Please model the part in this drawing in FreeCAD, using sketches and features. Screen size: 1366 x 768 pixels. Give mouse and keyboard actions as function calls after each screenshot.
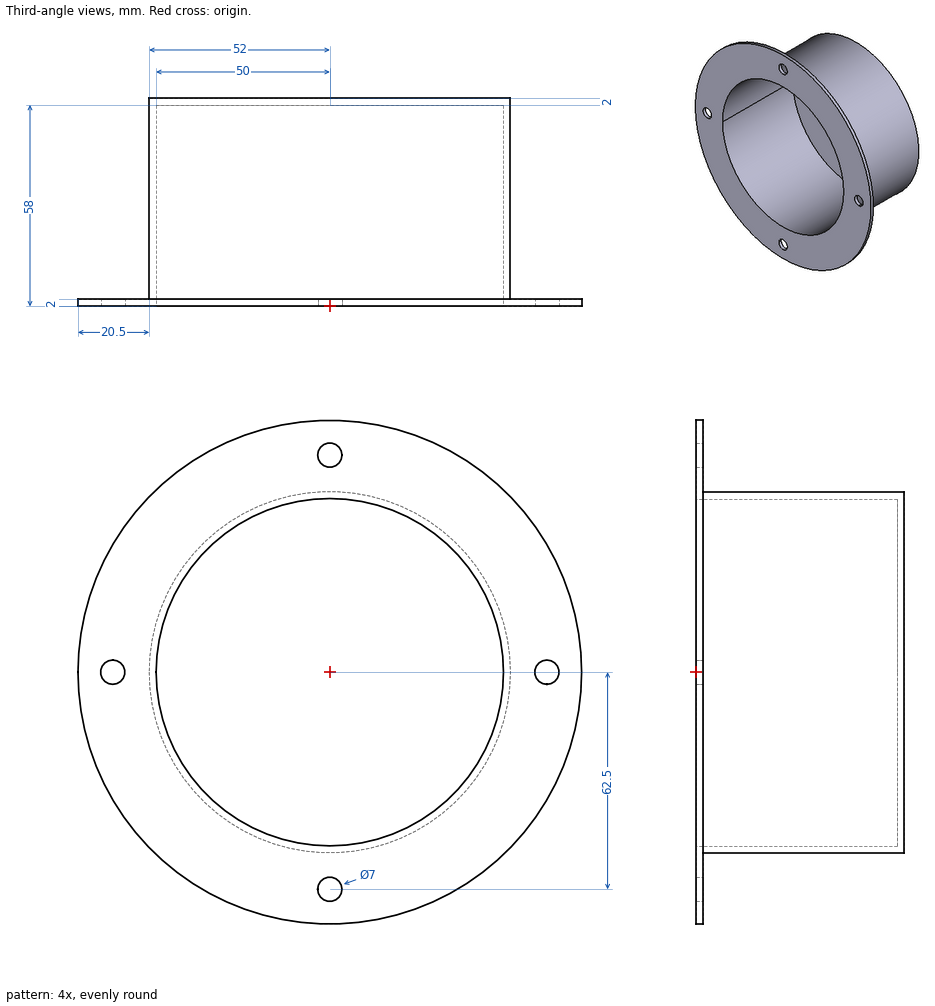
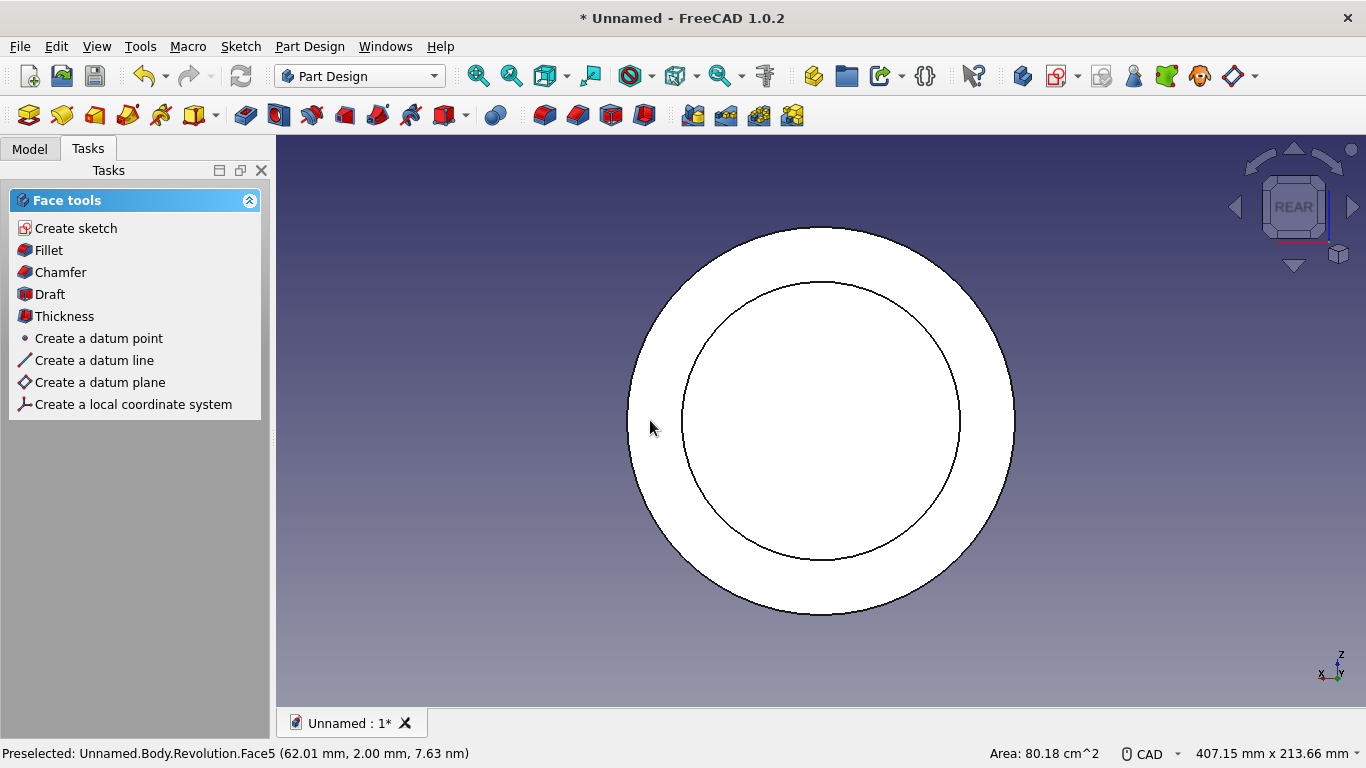
click(1056, 76)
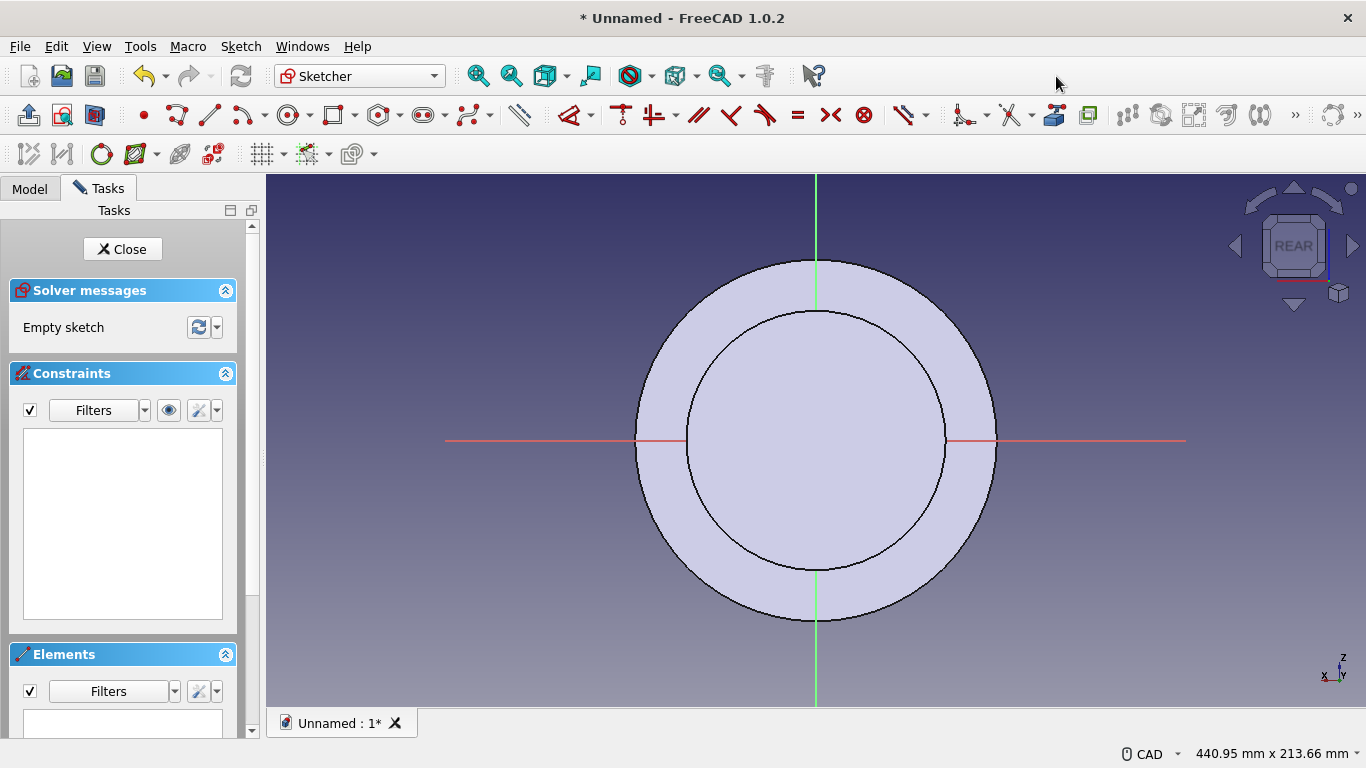
key(q)
key(s)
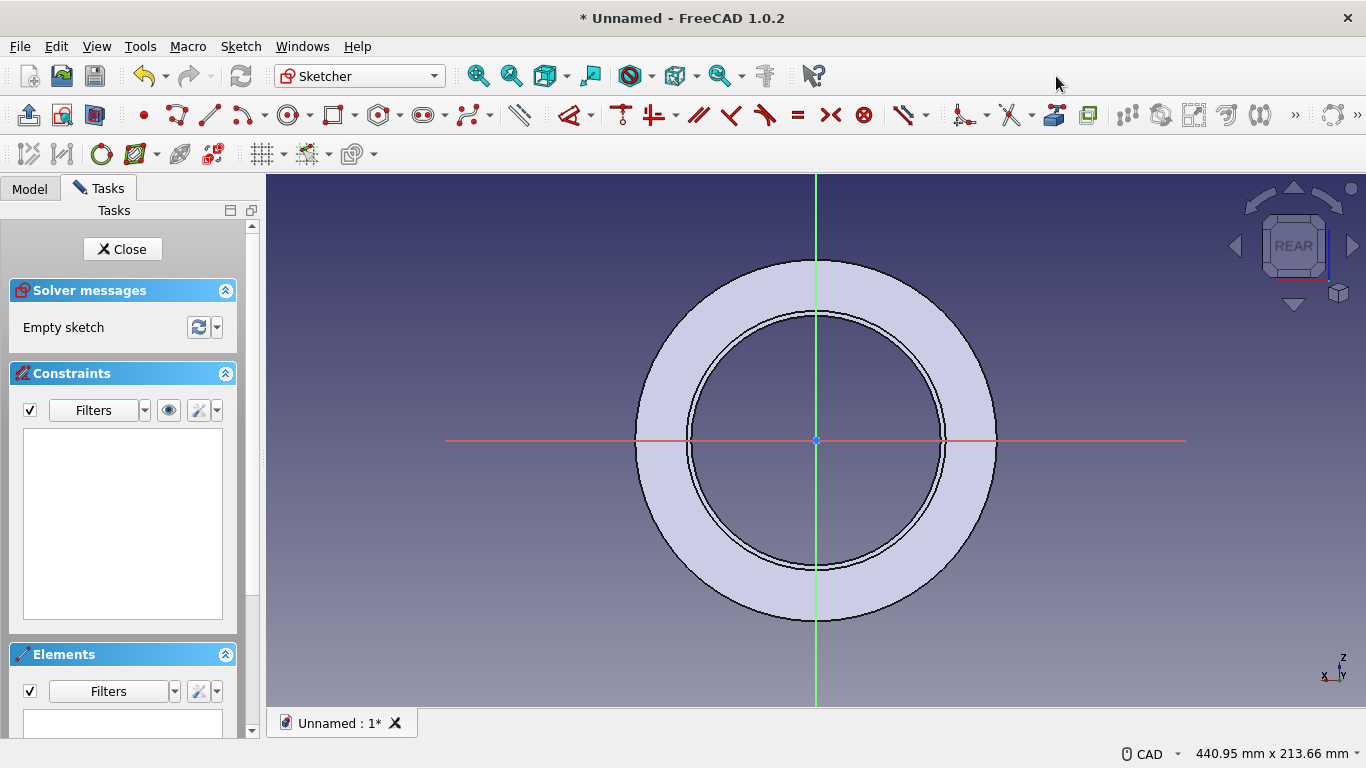
scroll(820, 605, up, 15)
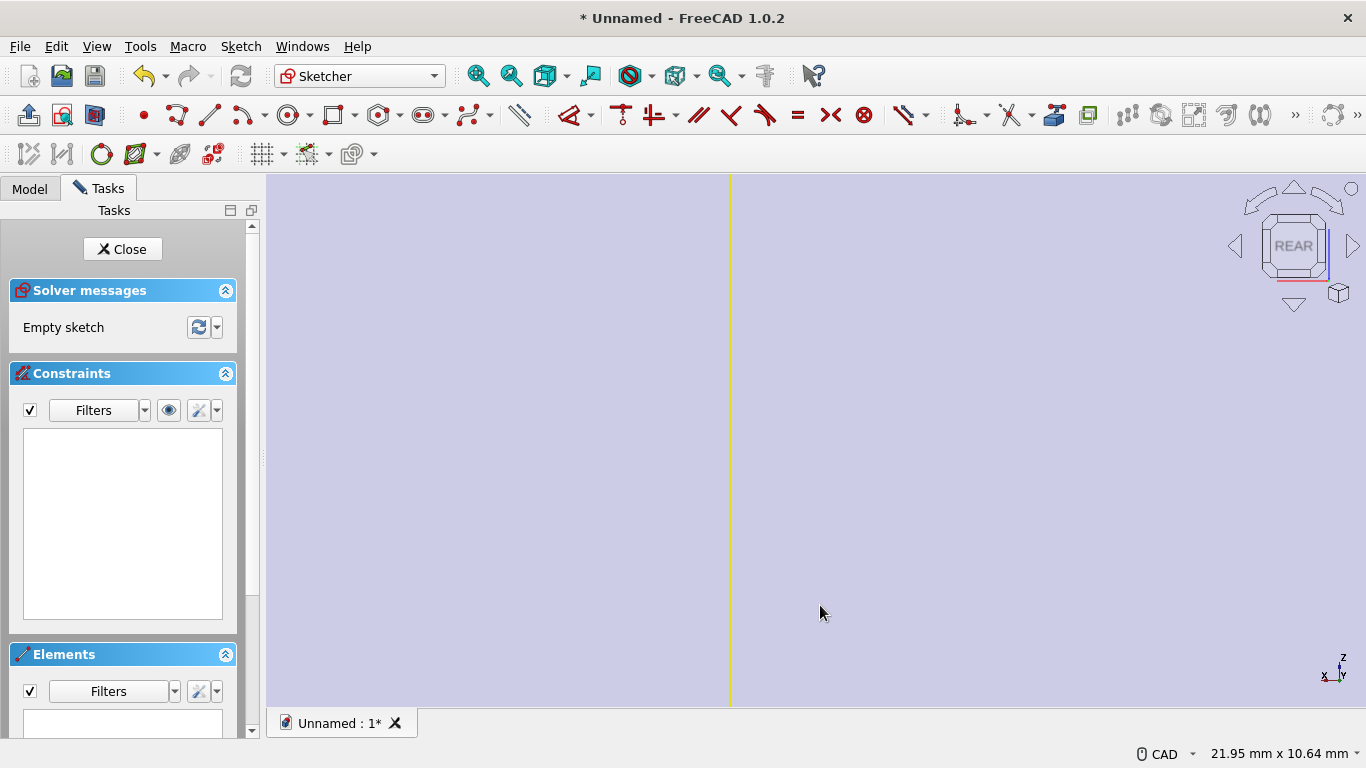
key(g)
key(c)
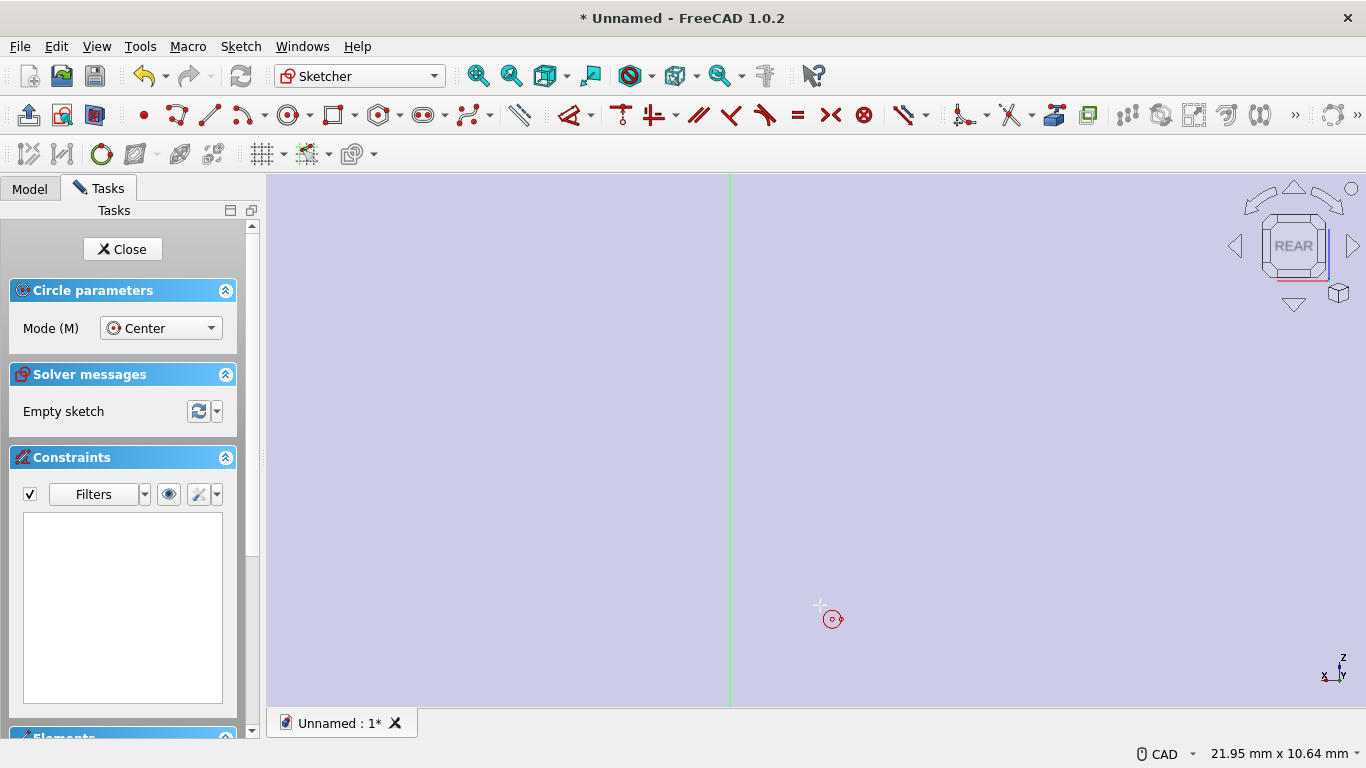
click(730, 417)
move(854, 293)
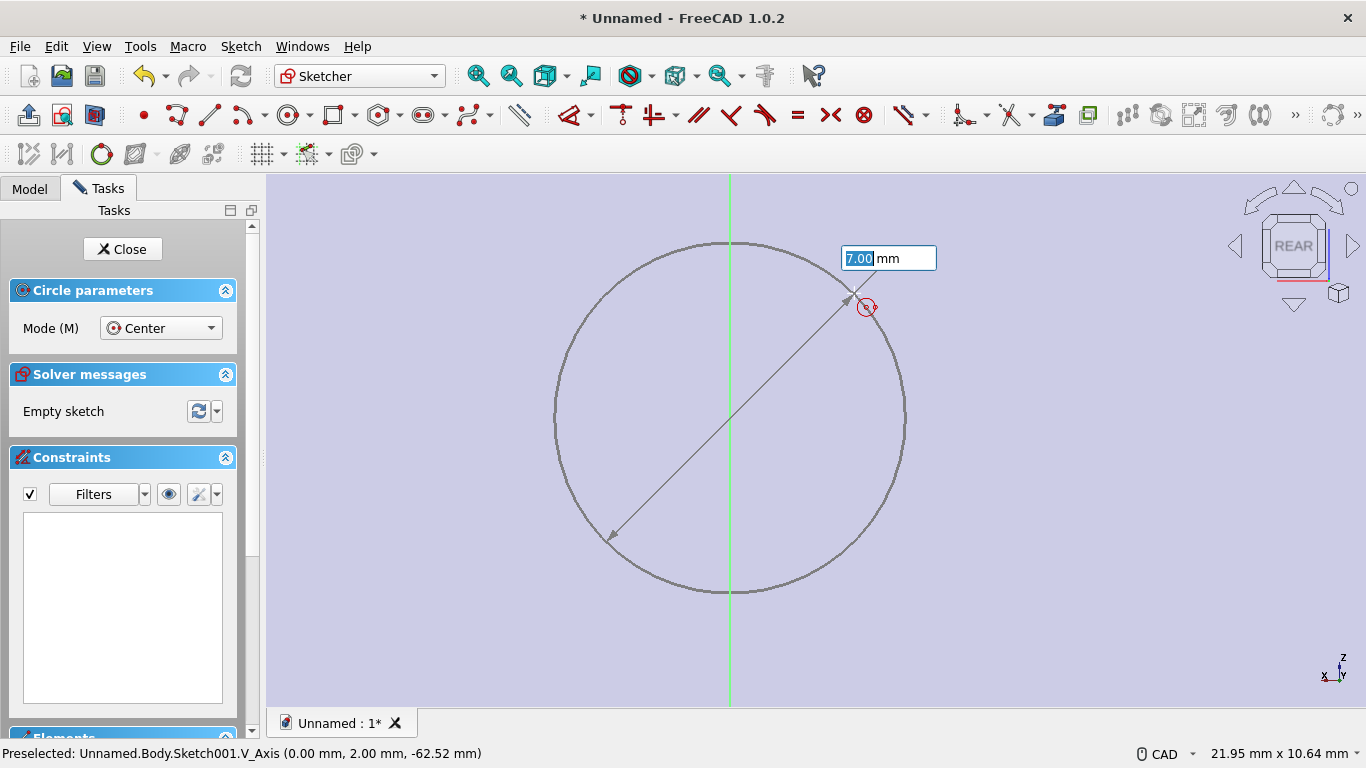
text(7)
key(Return)
key(Escape)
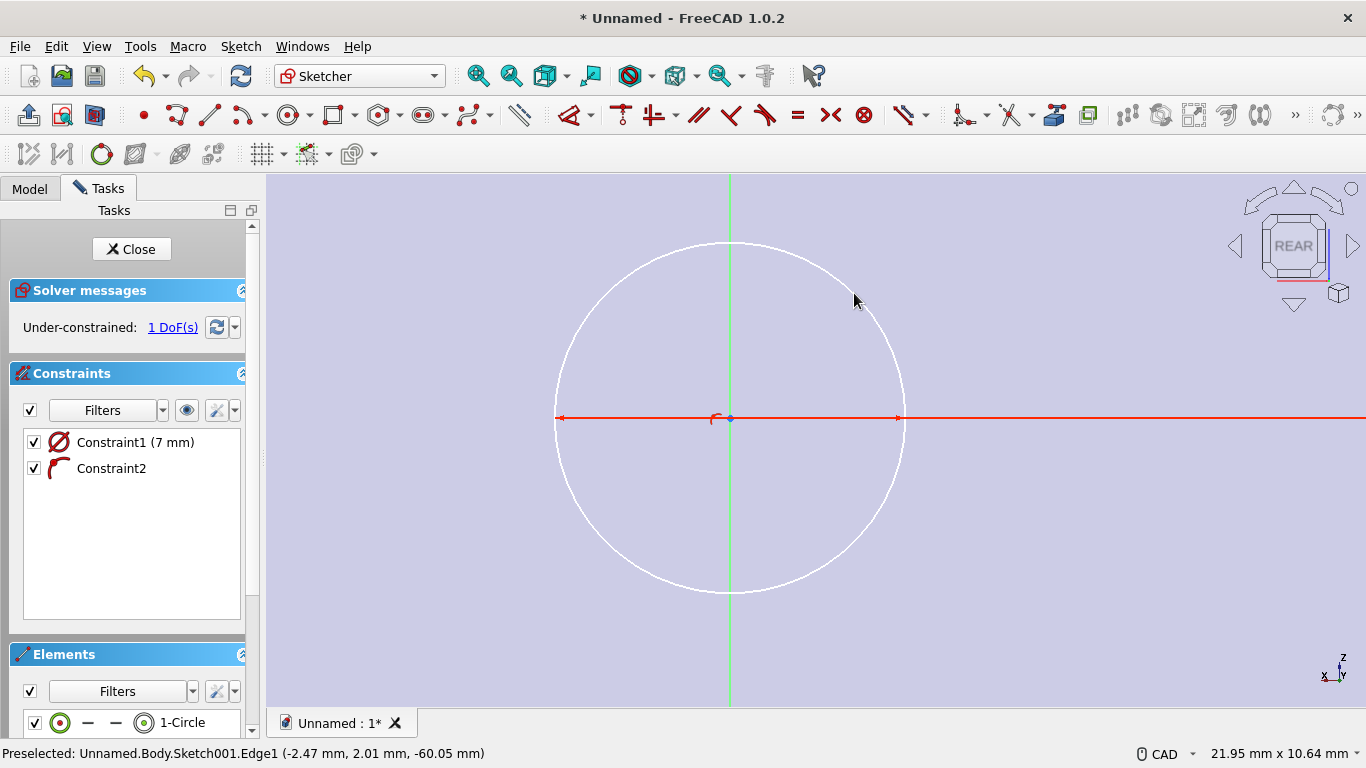
key(d)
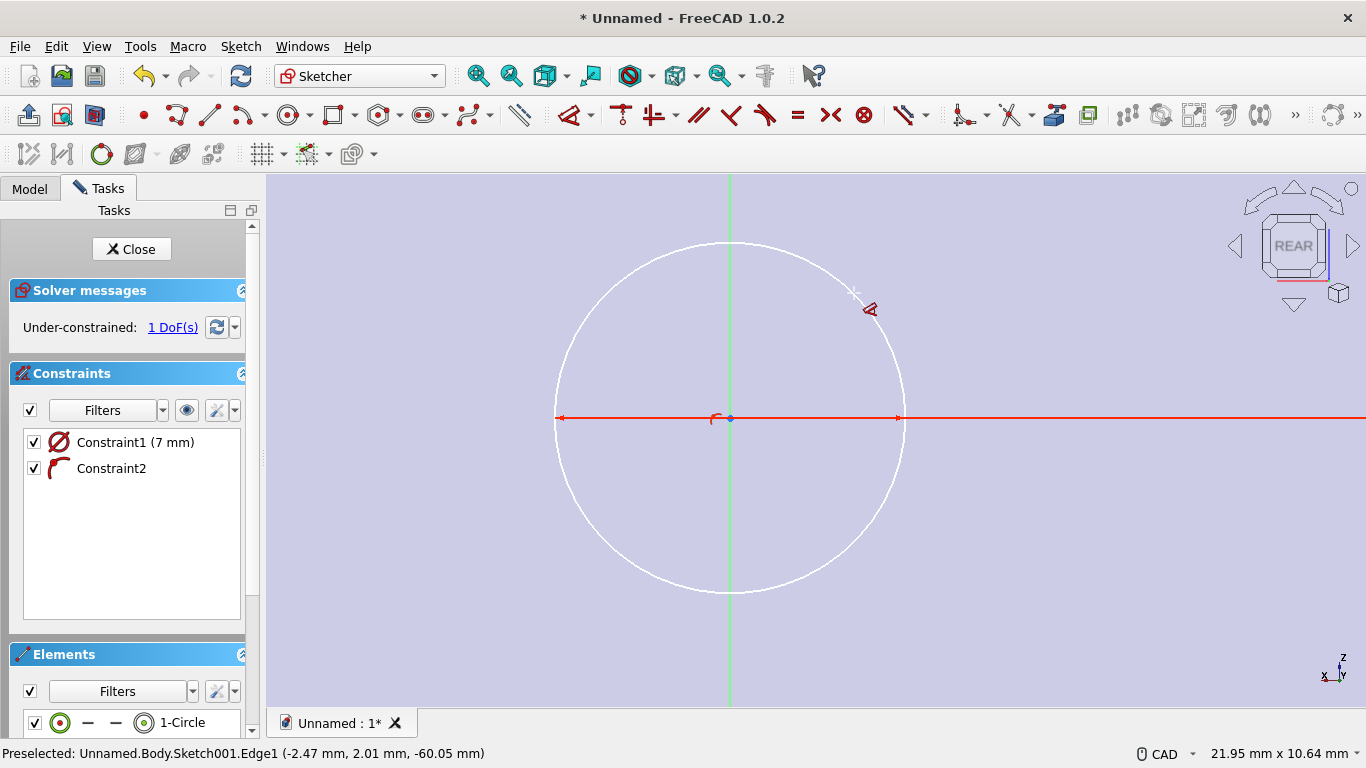
click(730, 418)
click(764, 310)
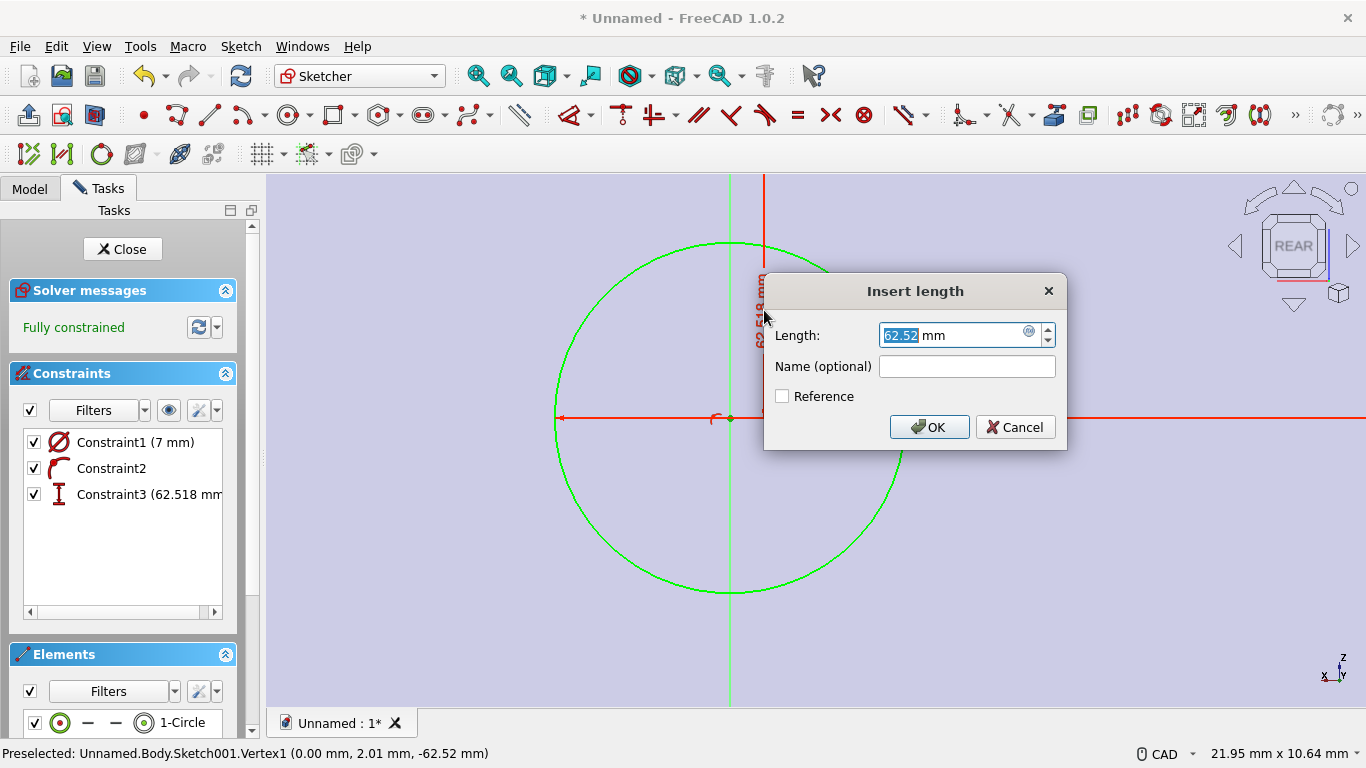
text(62.5)
key(Return)
key(Escape)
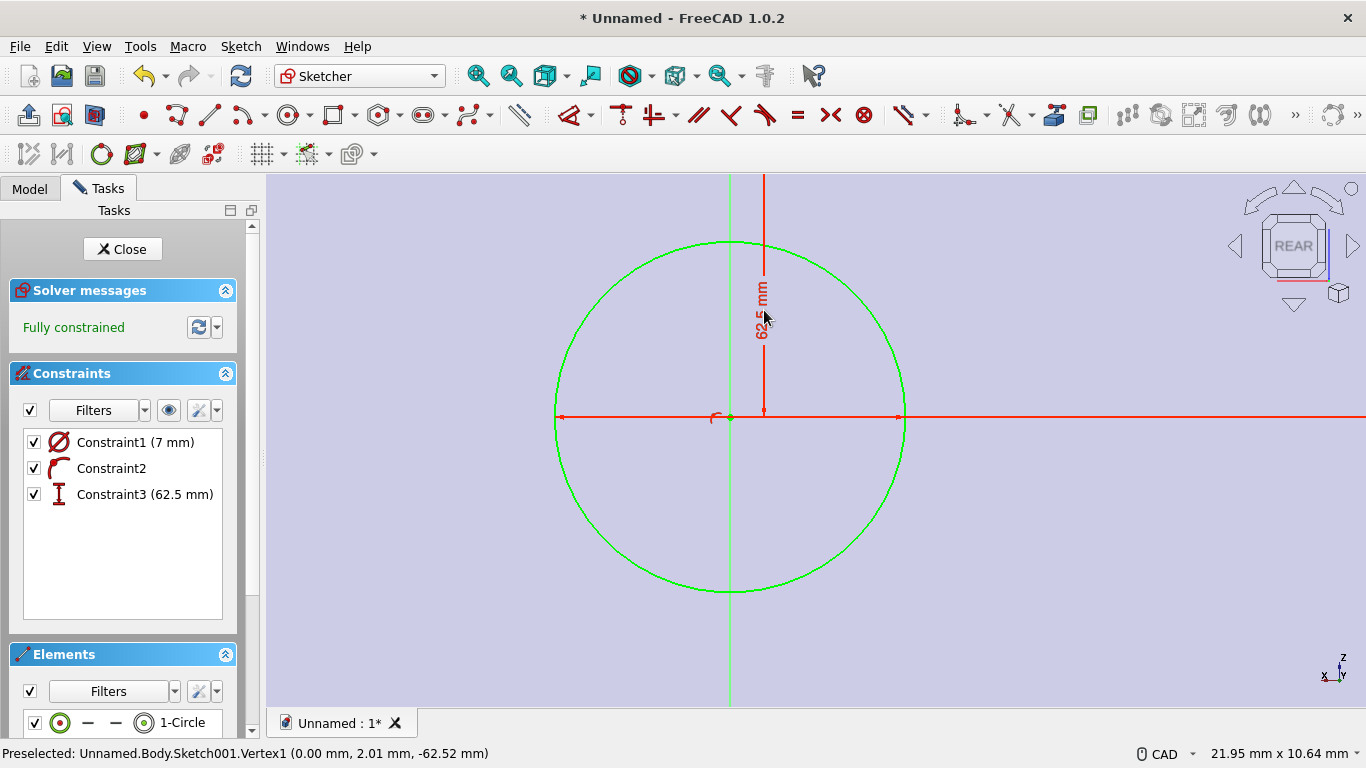
click(123, 249)